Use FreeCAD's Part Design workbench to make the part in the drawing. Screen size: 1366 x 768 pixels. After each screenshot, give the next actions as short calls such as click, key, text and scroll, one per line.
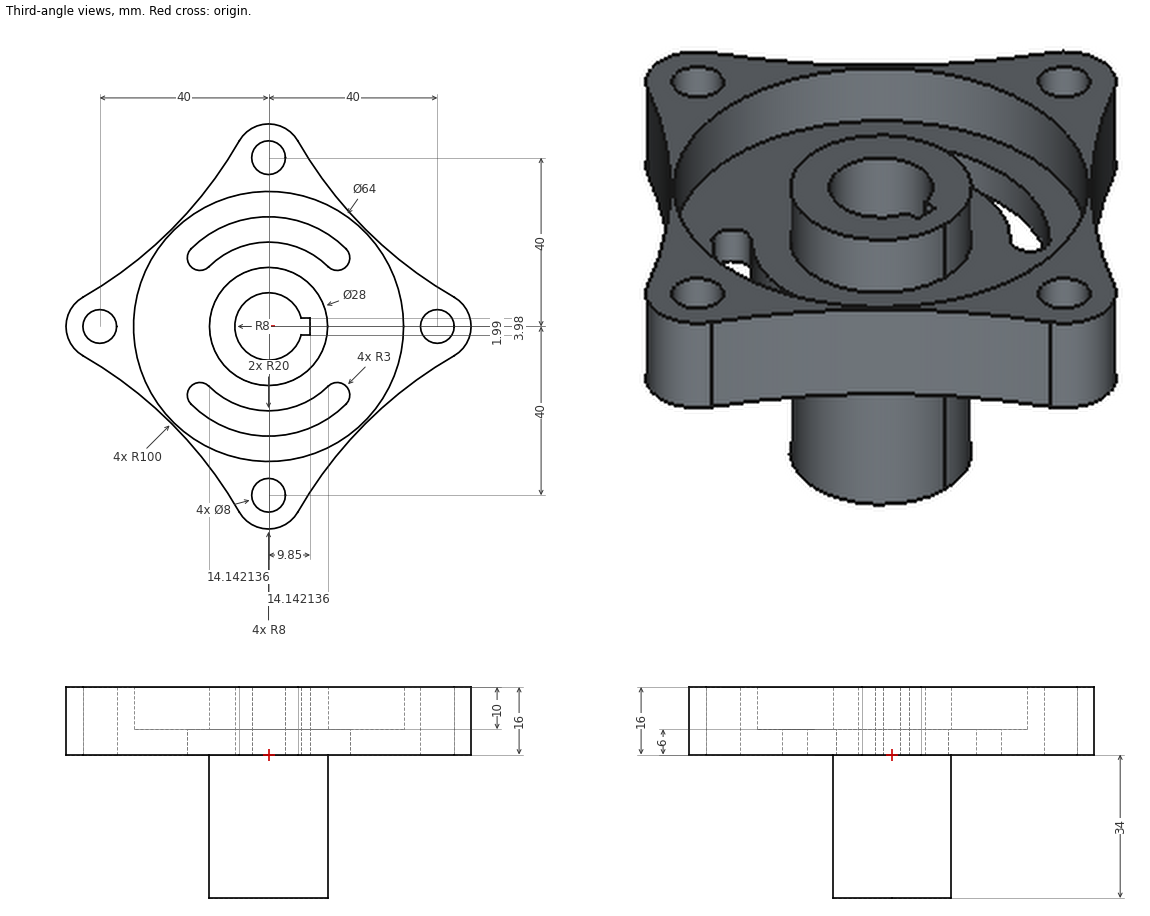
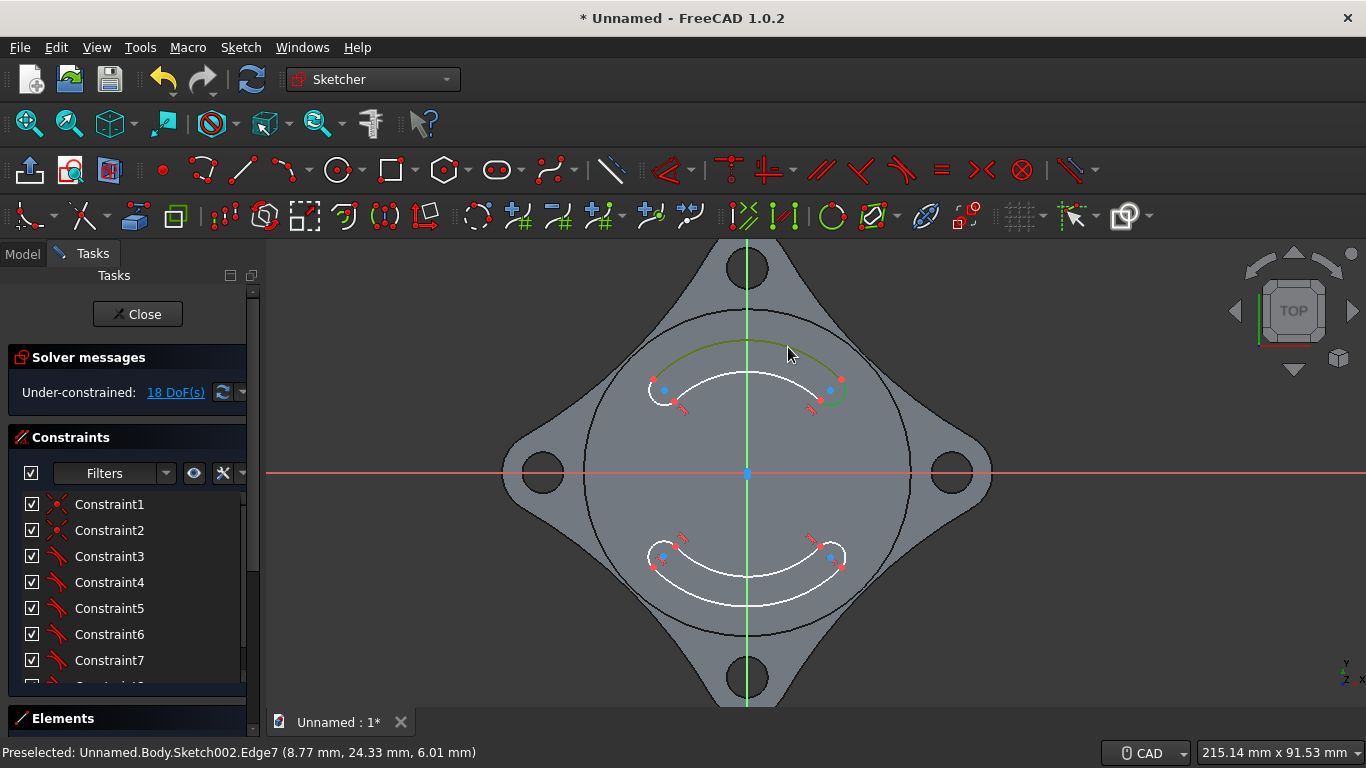
click(902, 170)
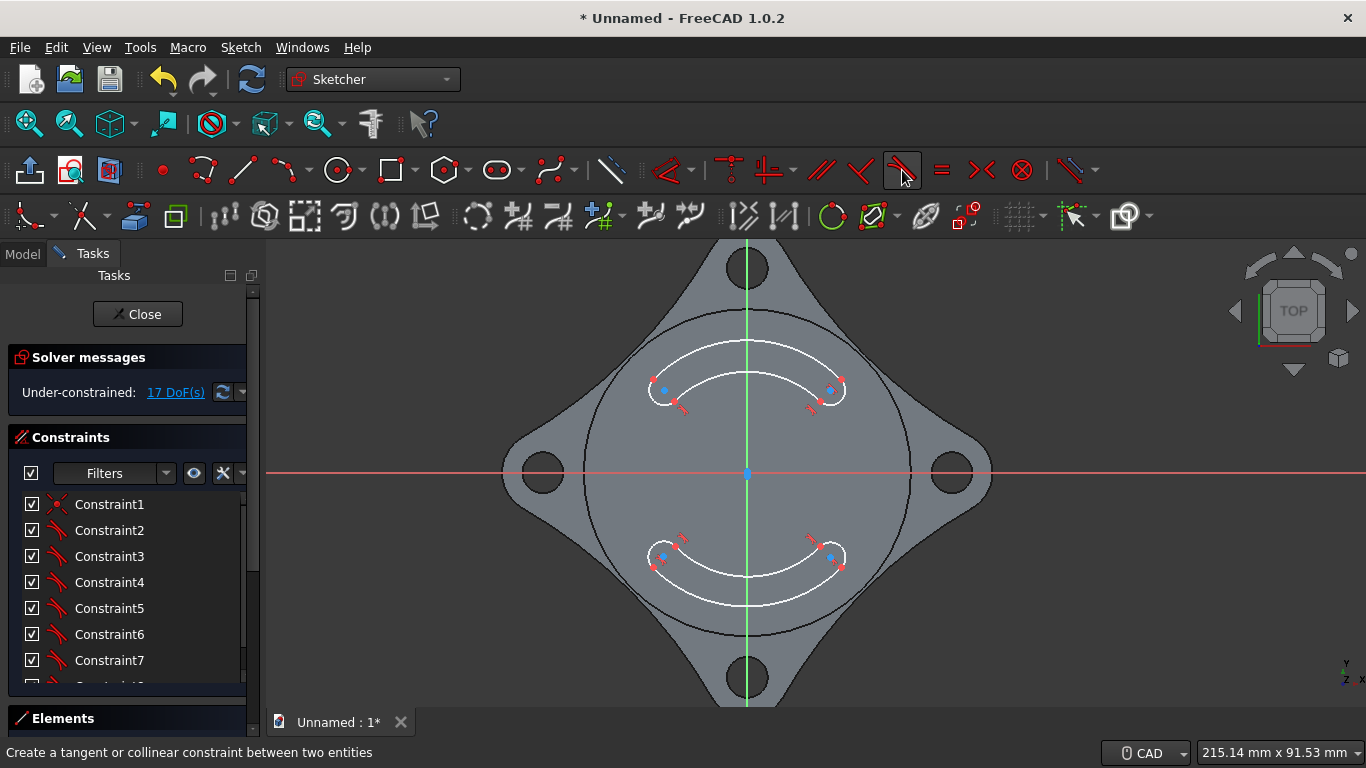
click(788, 347)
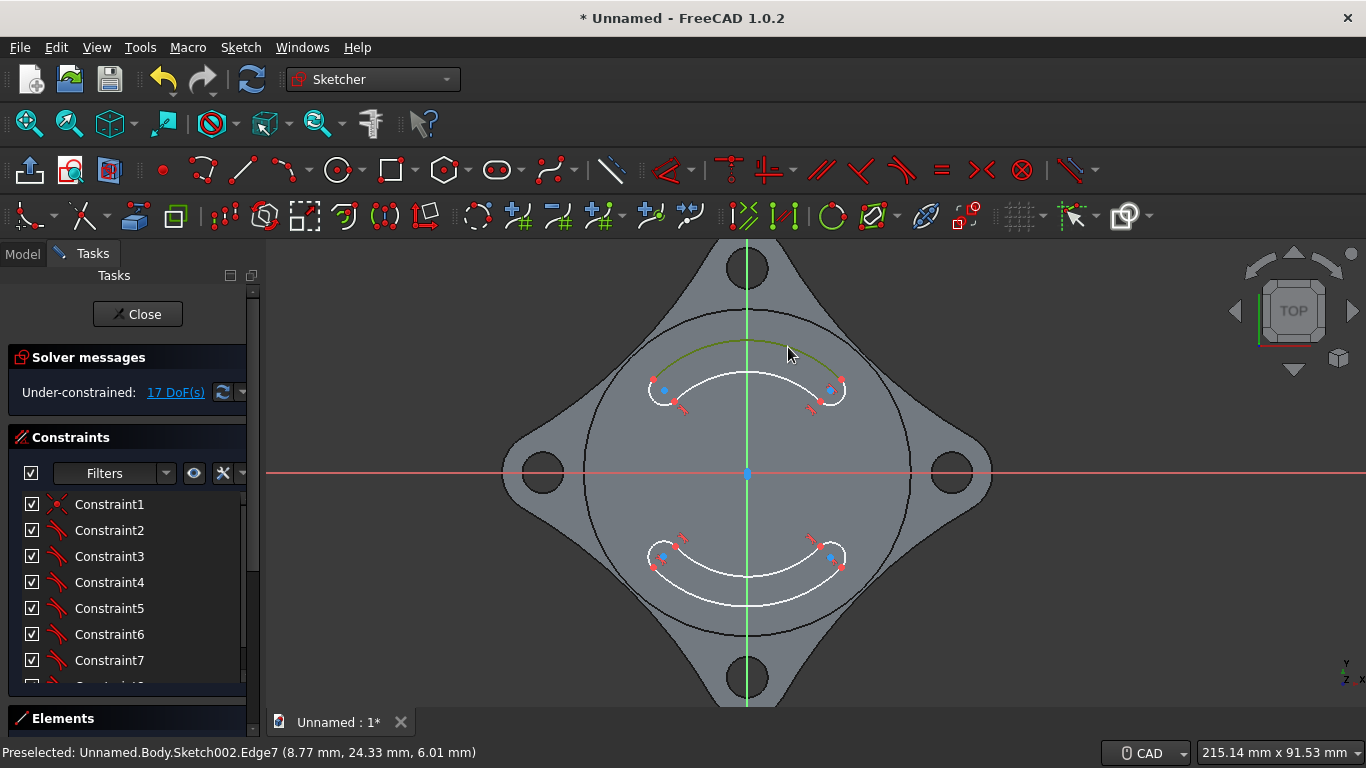
click(650, 393)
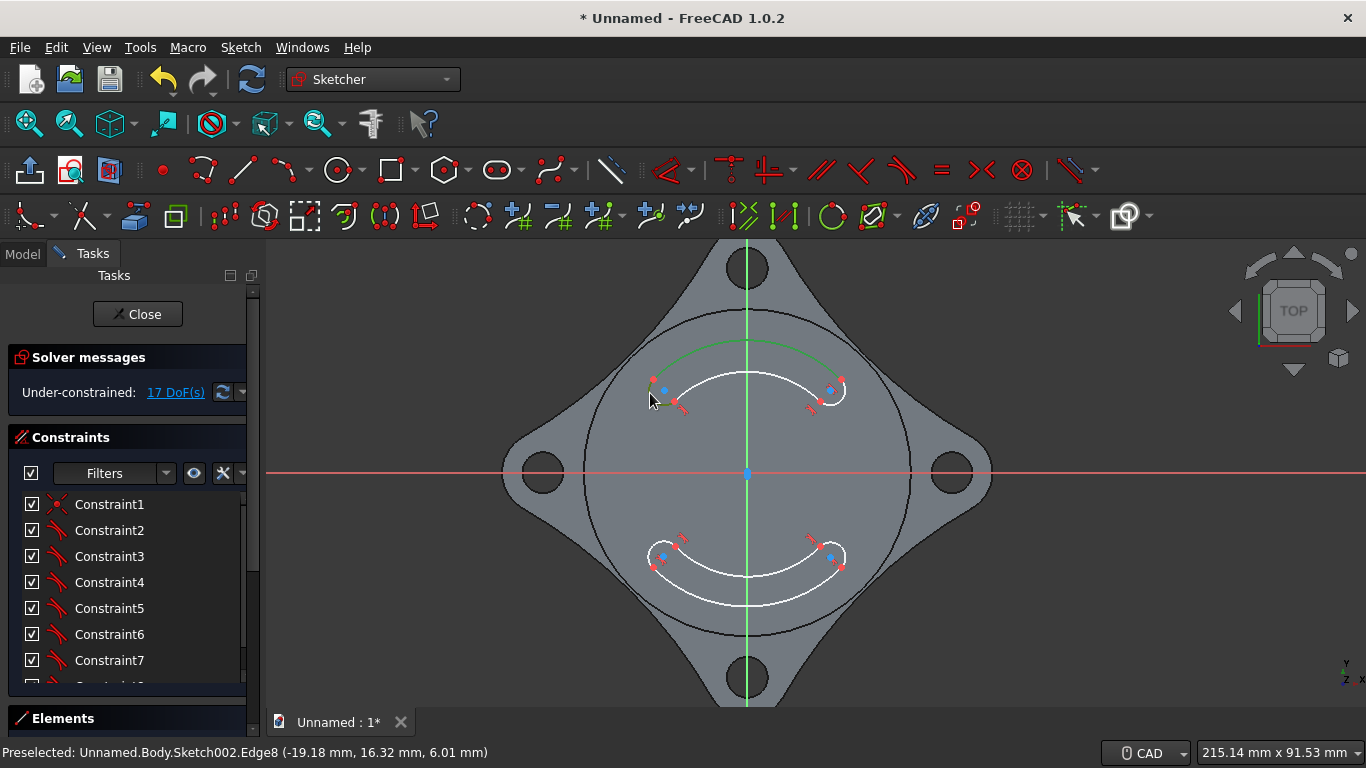
click(902, 170)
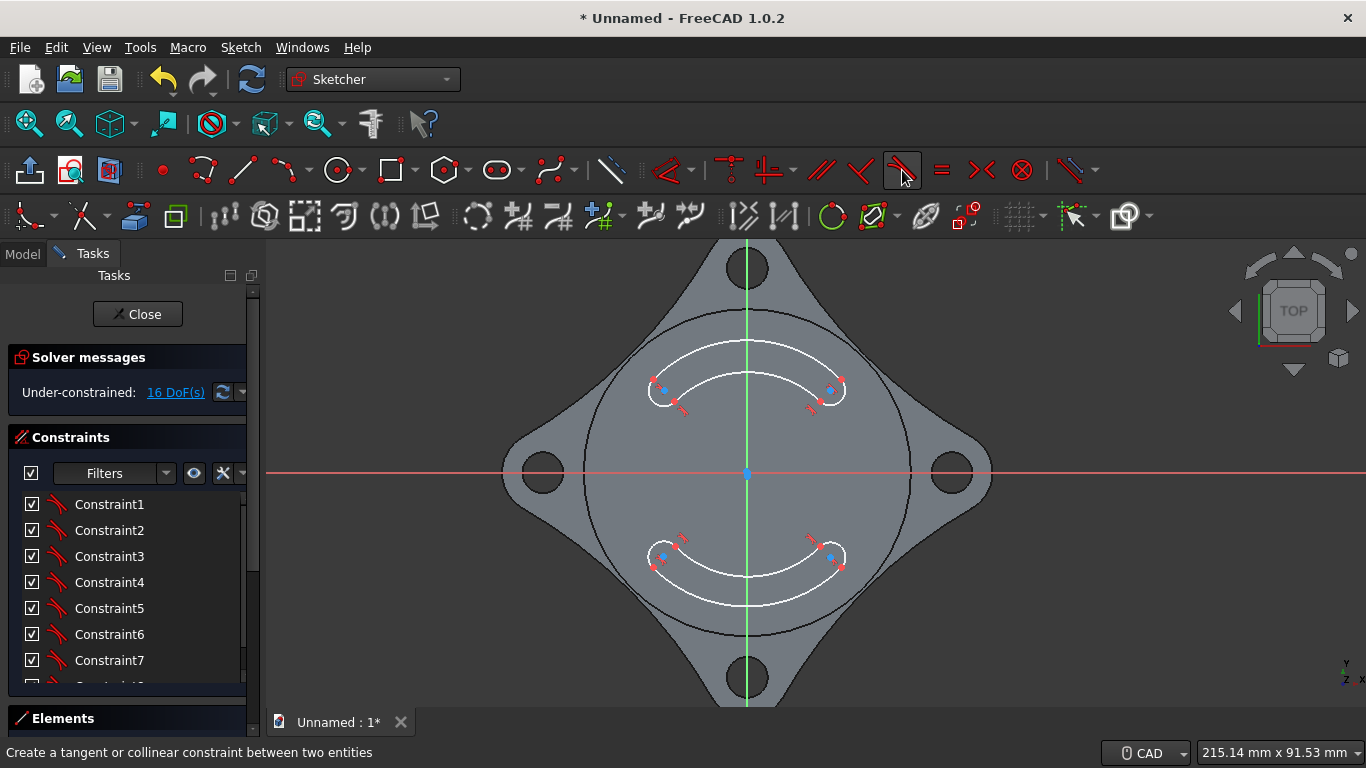
click(716, 571)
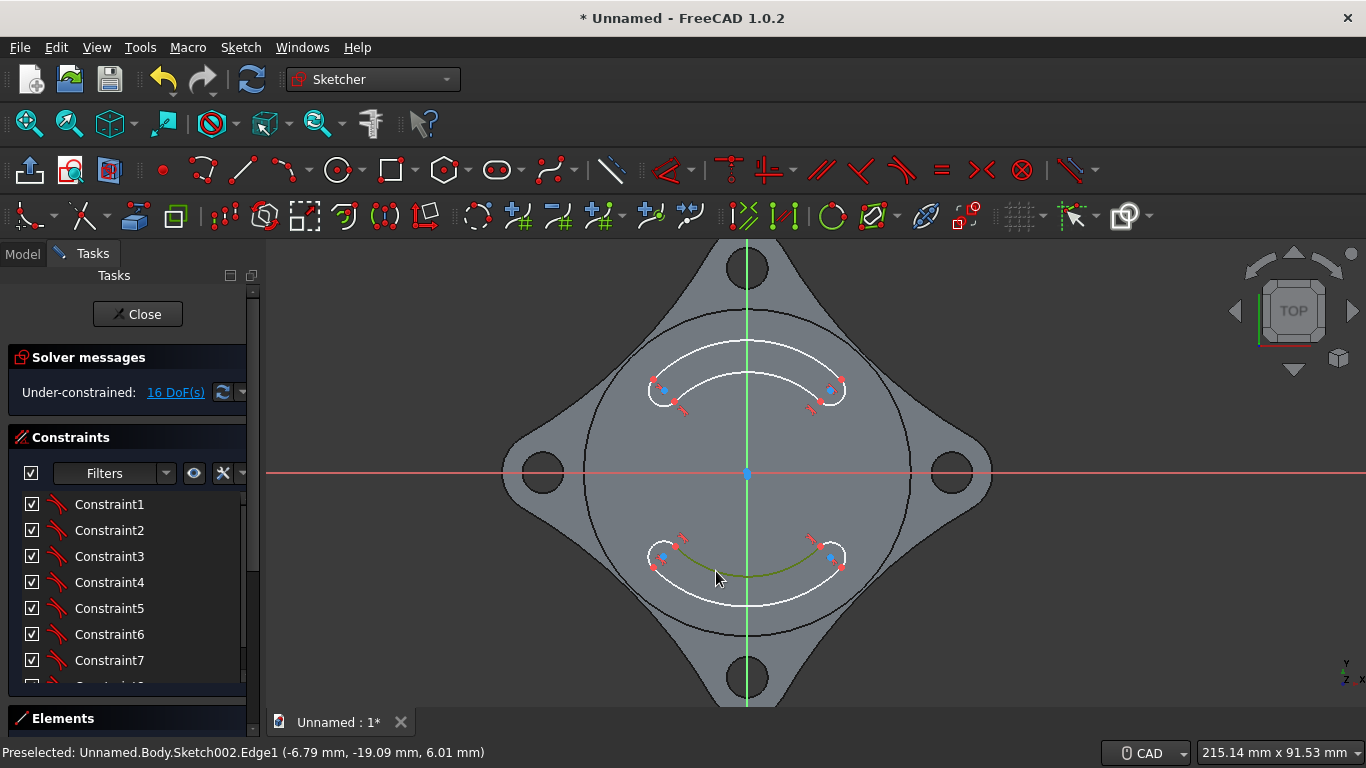
click(706, 600)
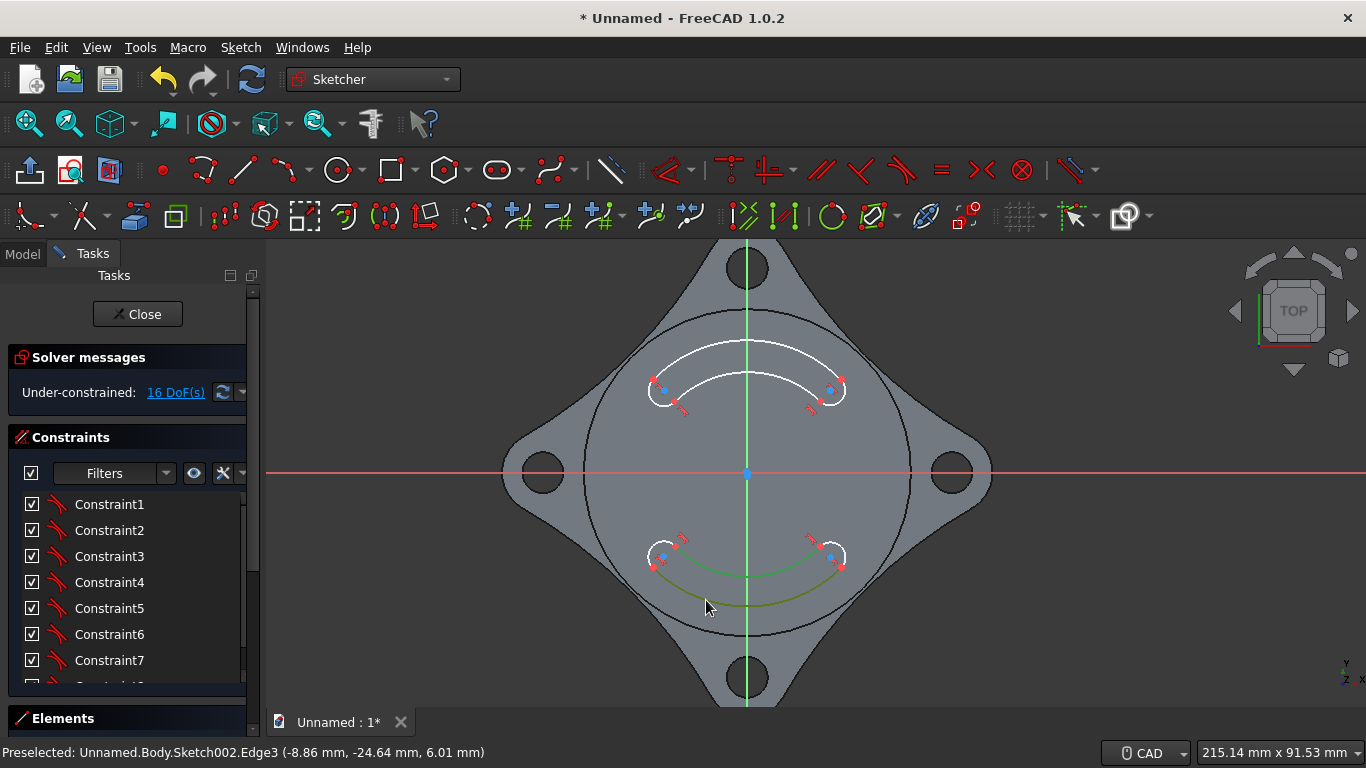
click(730, 170)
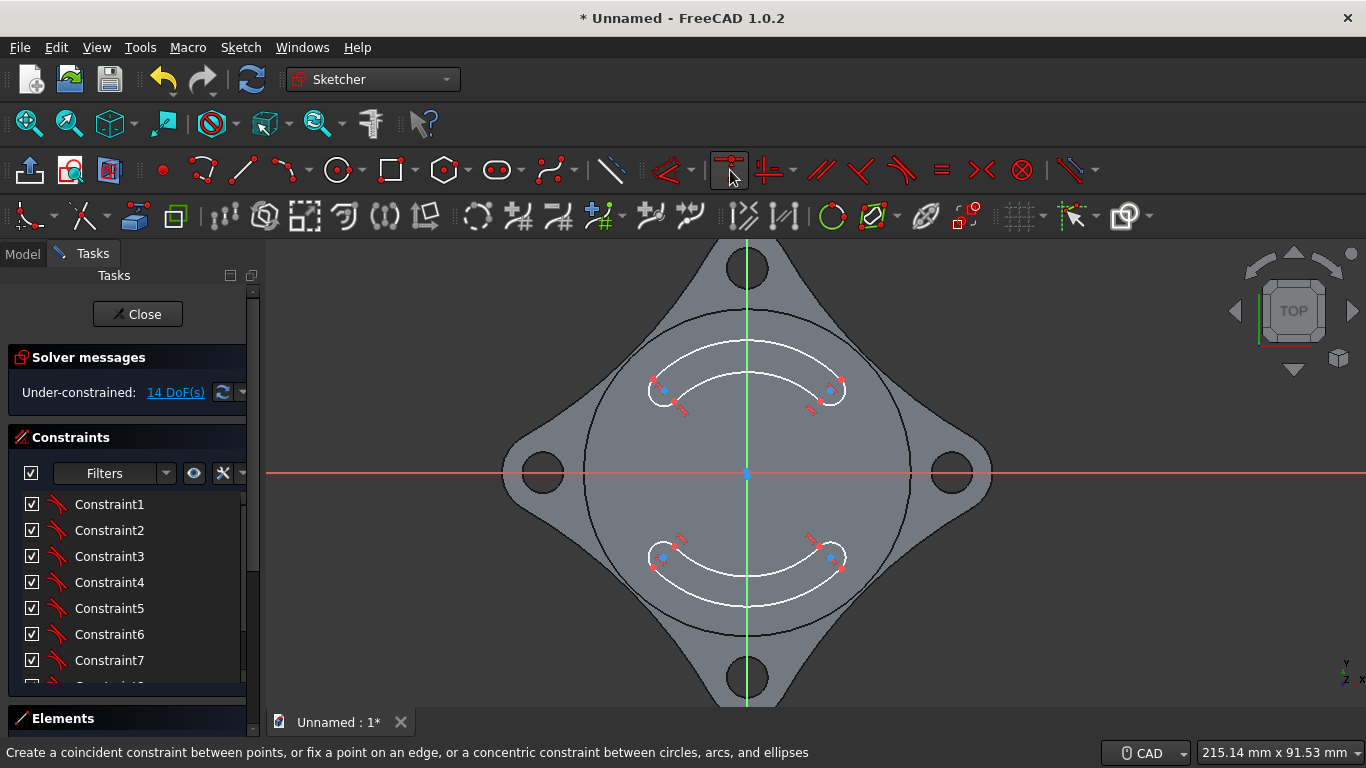
click(715, 571)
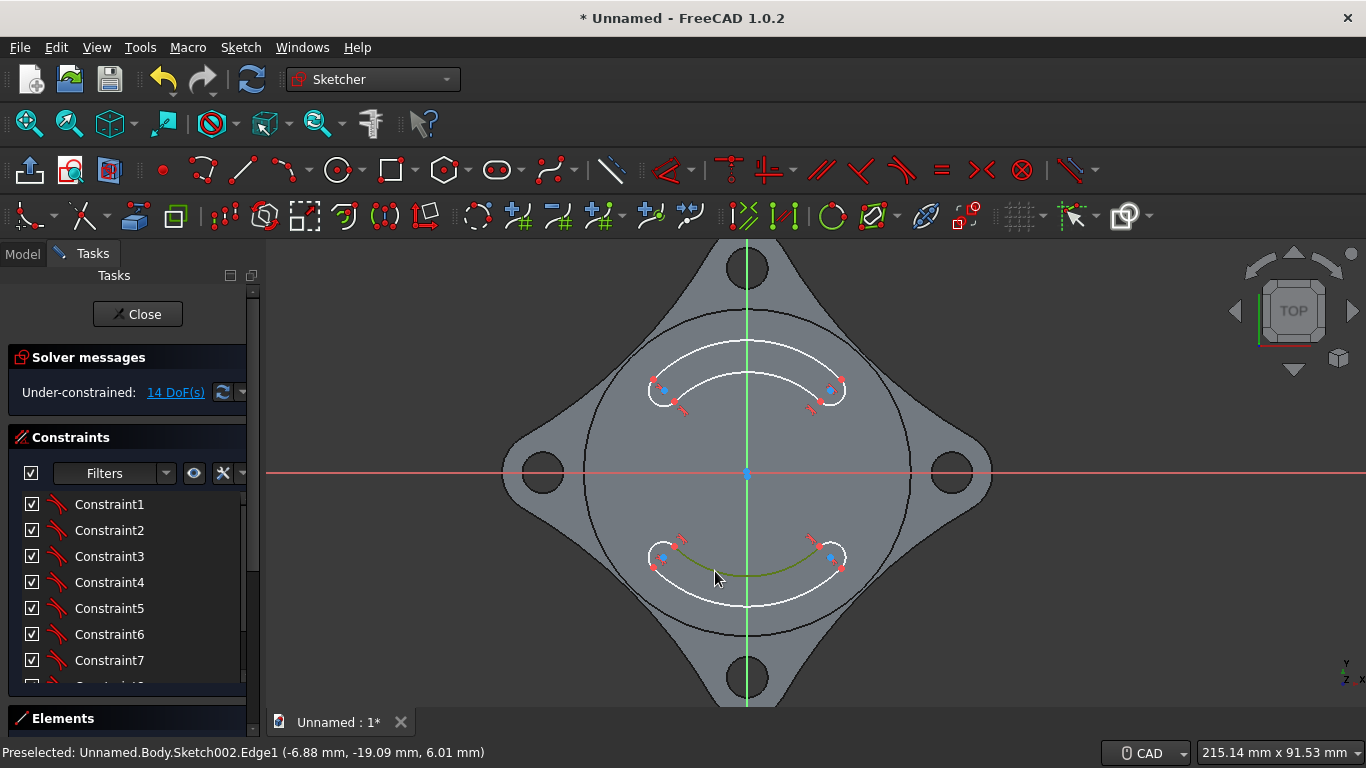
click(779, 377)